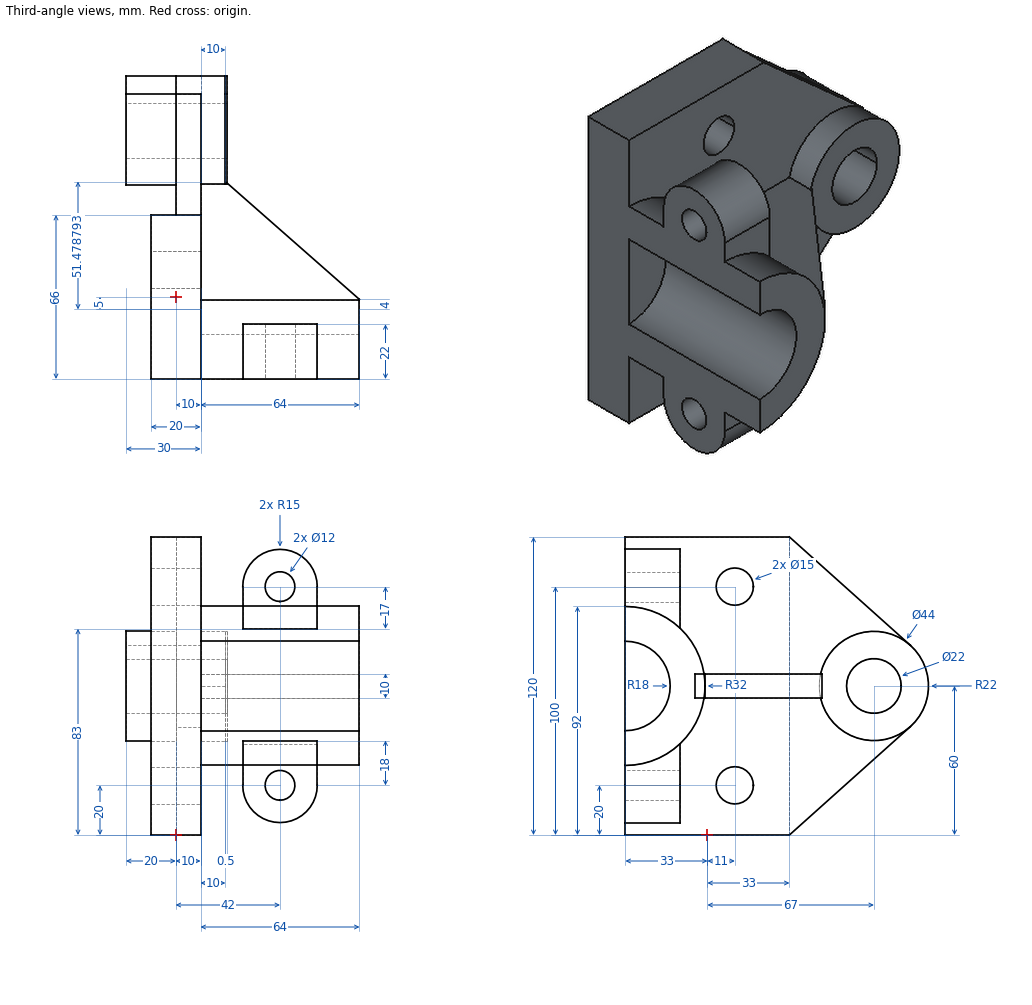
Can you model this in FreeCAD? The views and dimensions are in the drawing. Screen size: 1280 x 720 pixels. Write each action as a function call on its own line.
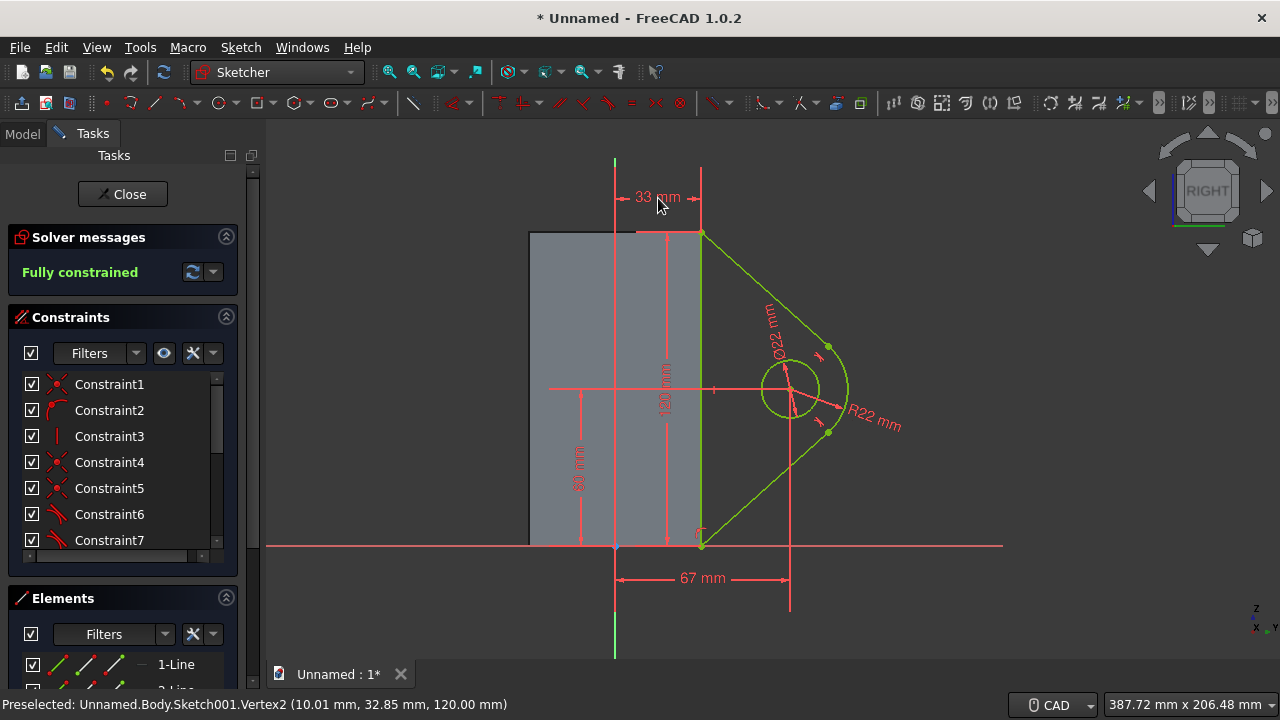
click(123, 194)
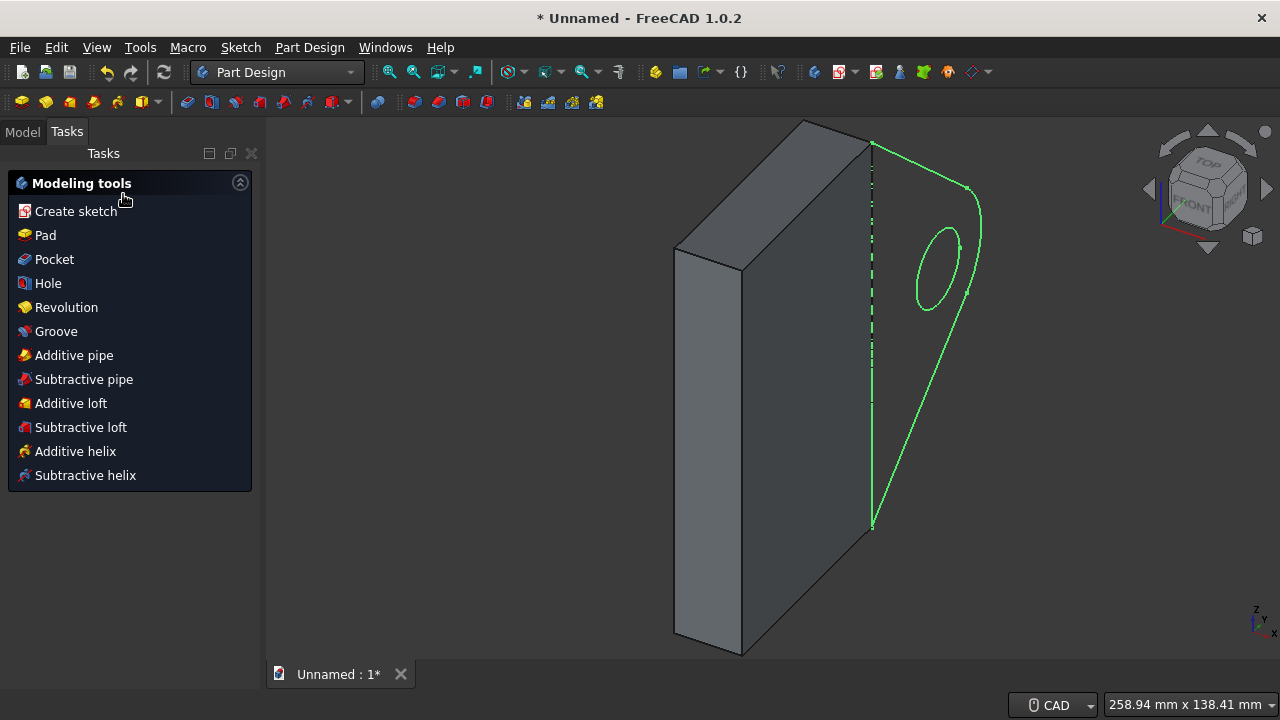
click(22, 102)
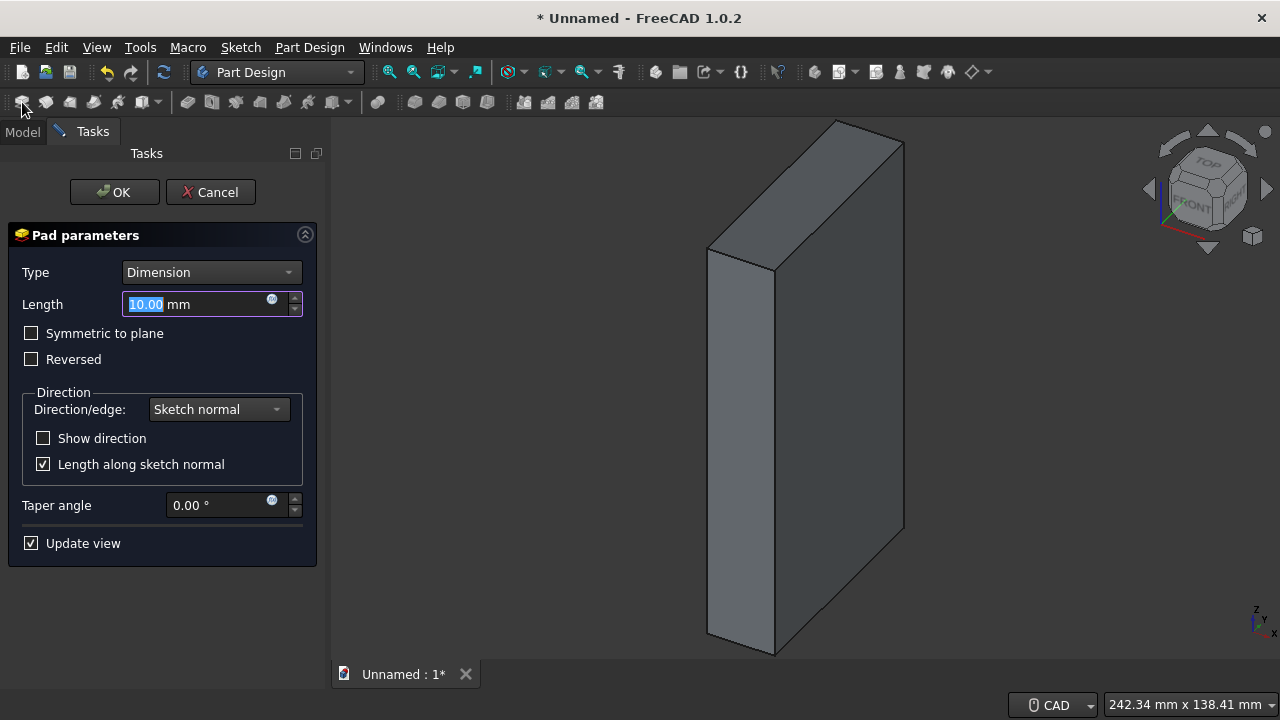
text(10)
key(Tab)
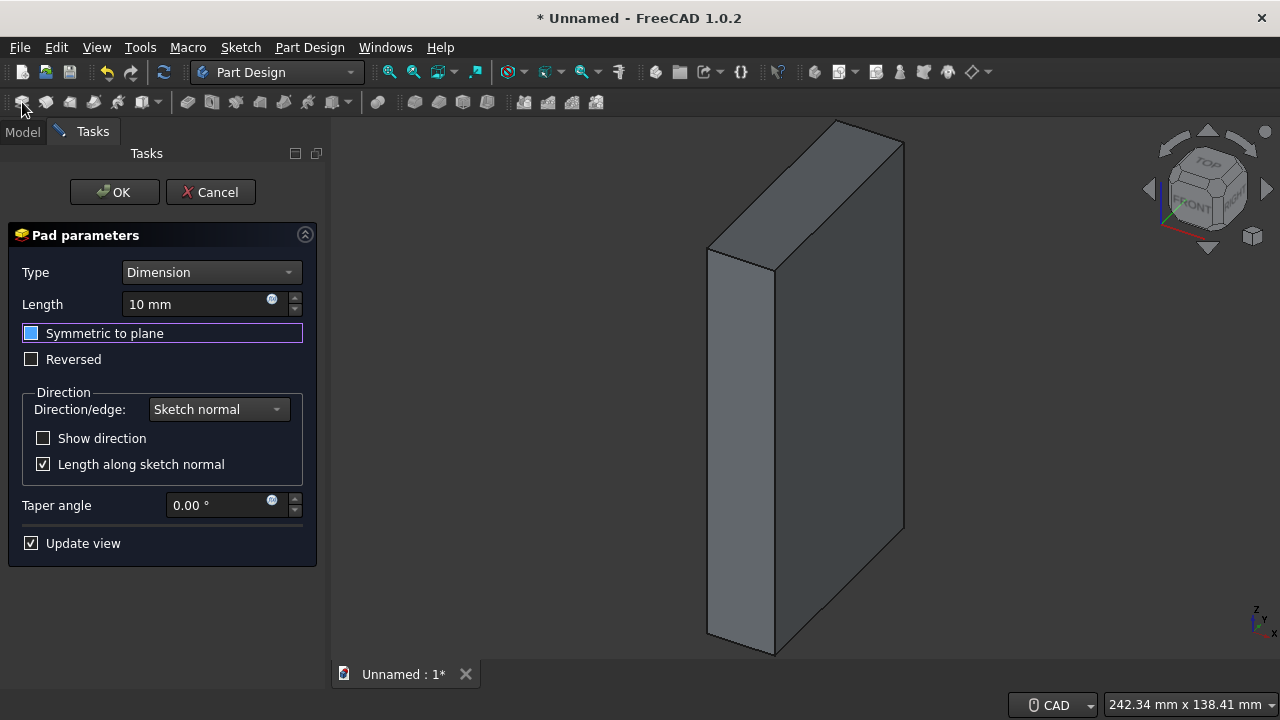
click(30, 359)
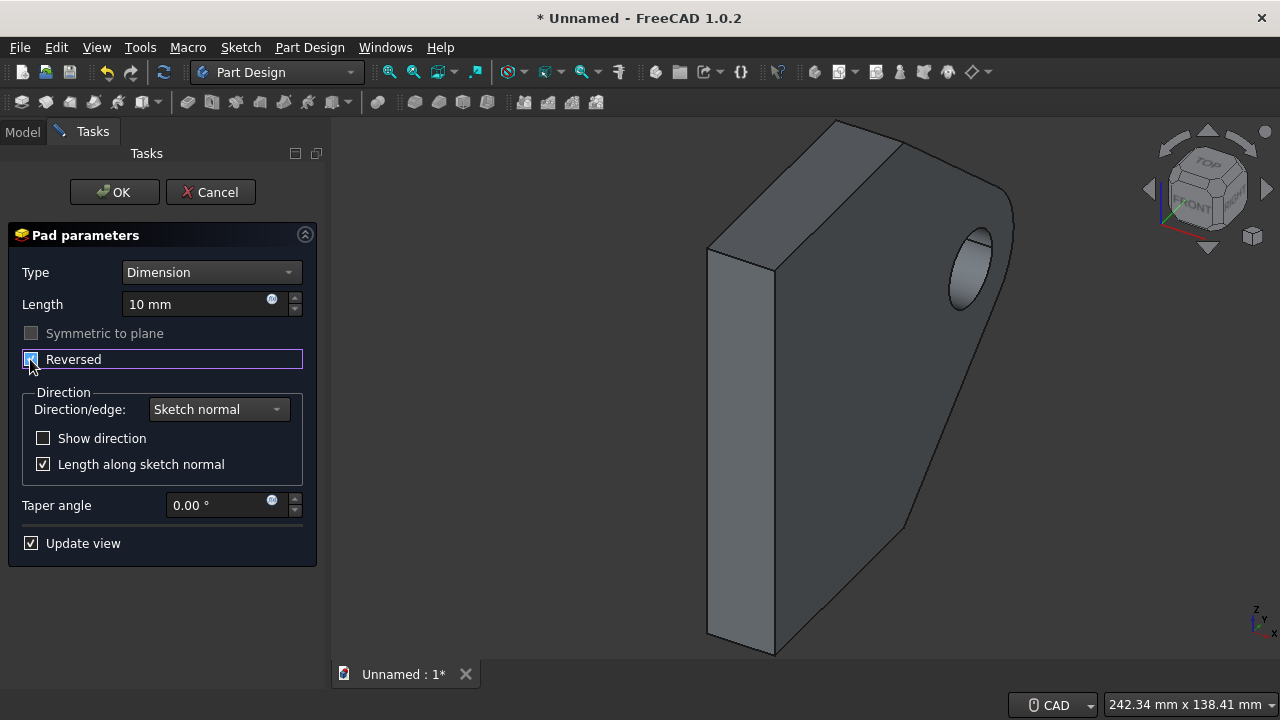
click(115, 192)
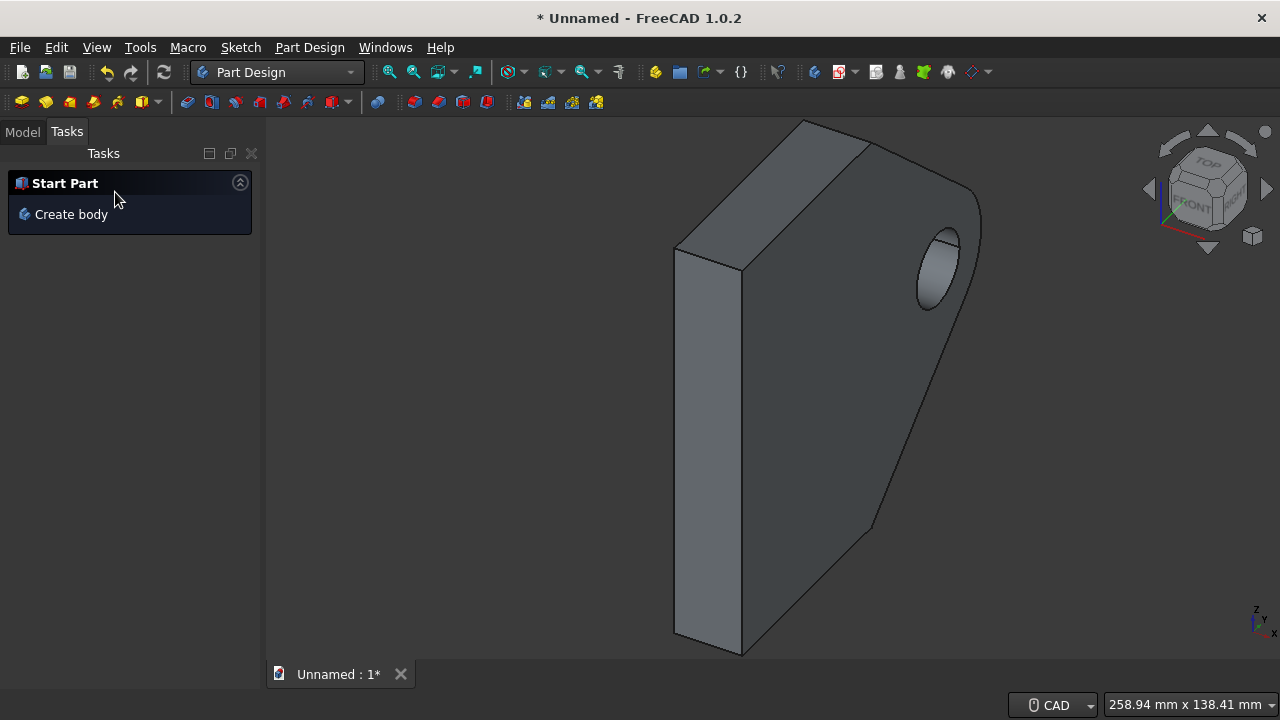
click(390, 72)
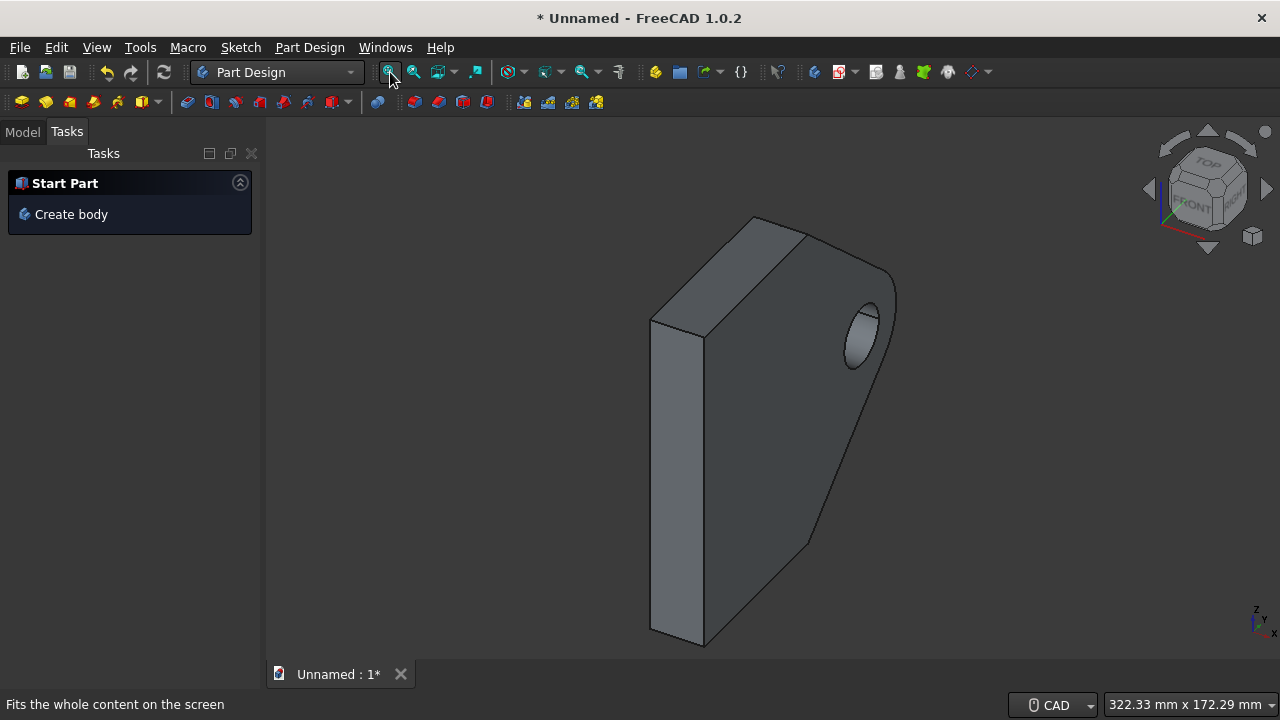
key(6)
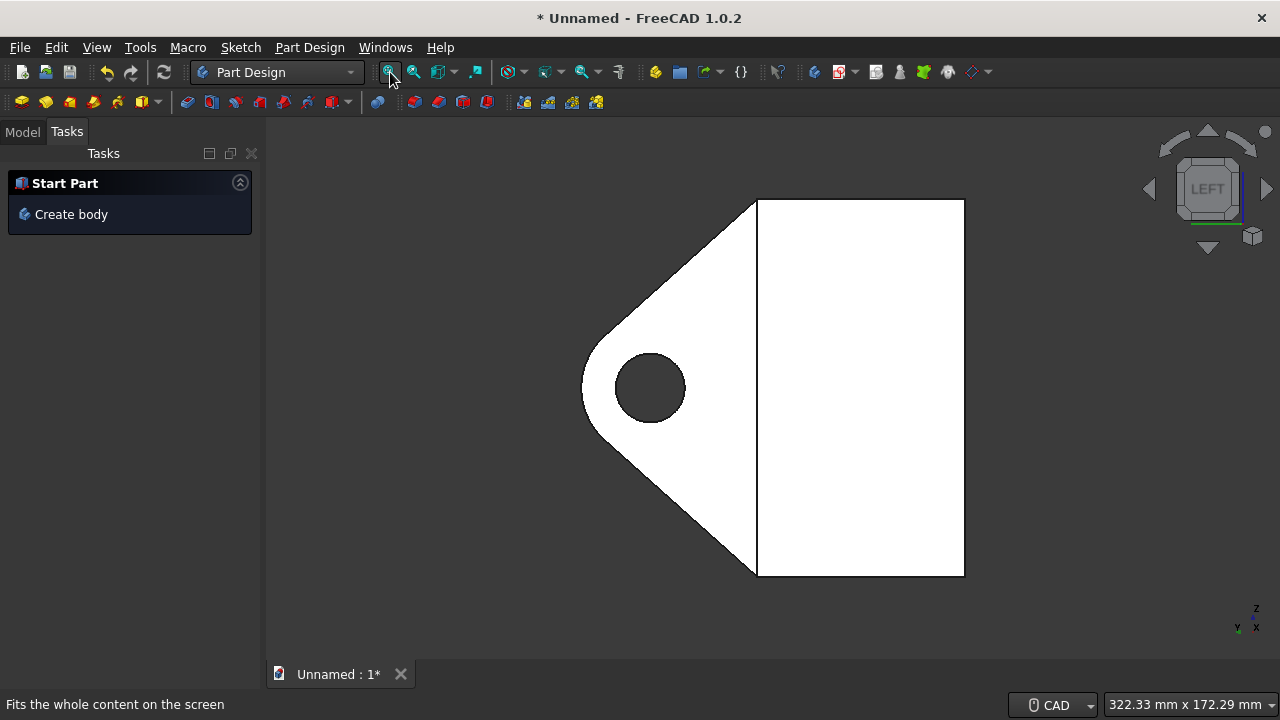
click(720, 333)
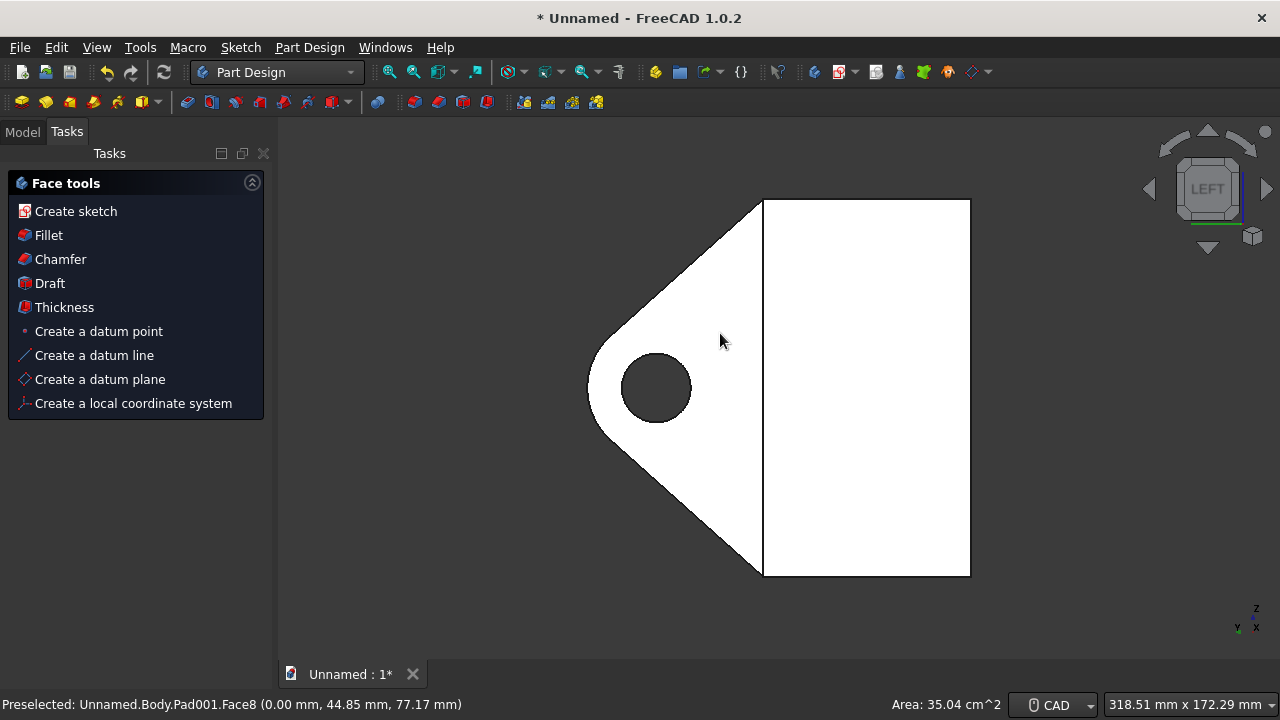
click(840, 72)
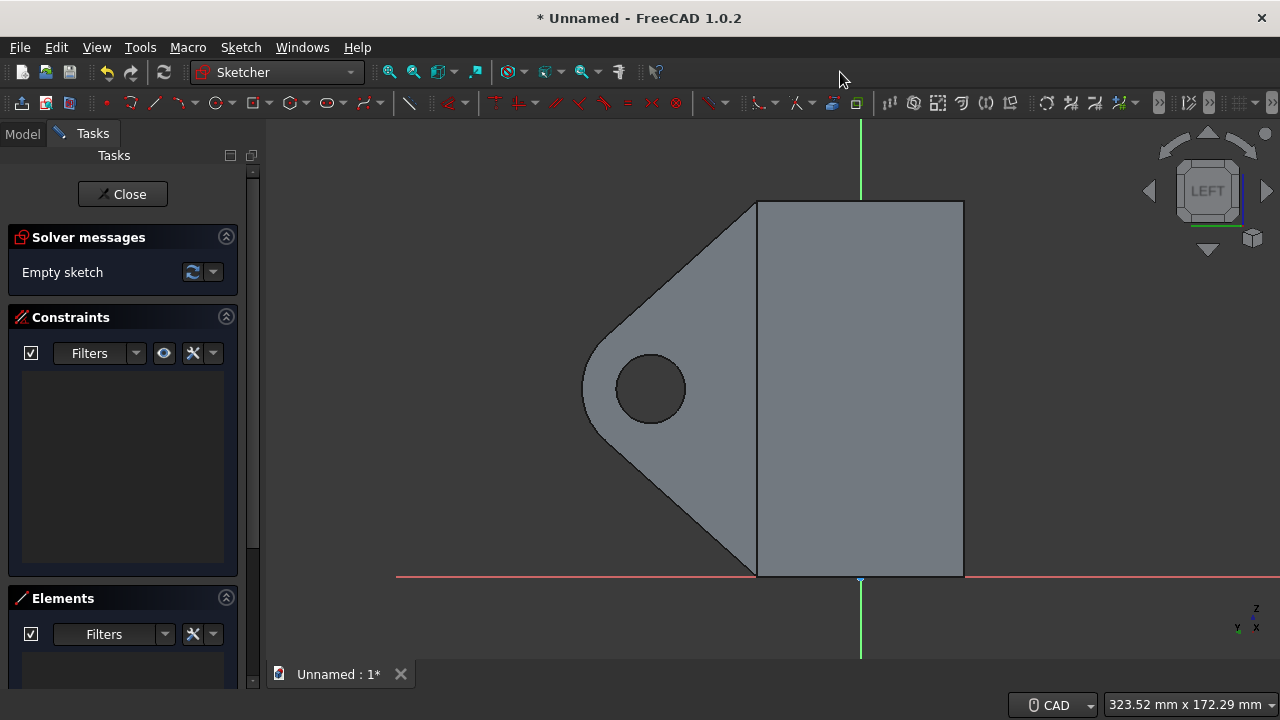
click(70, 104)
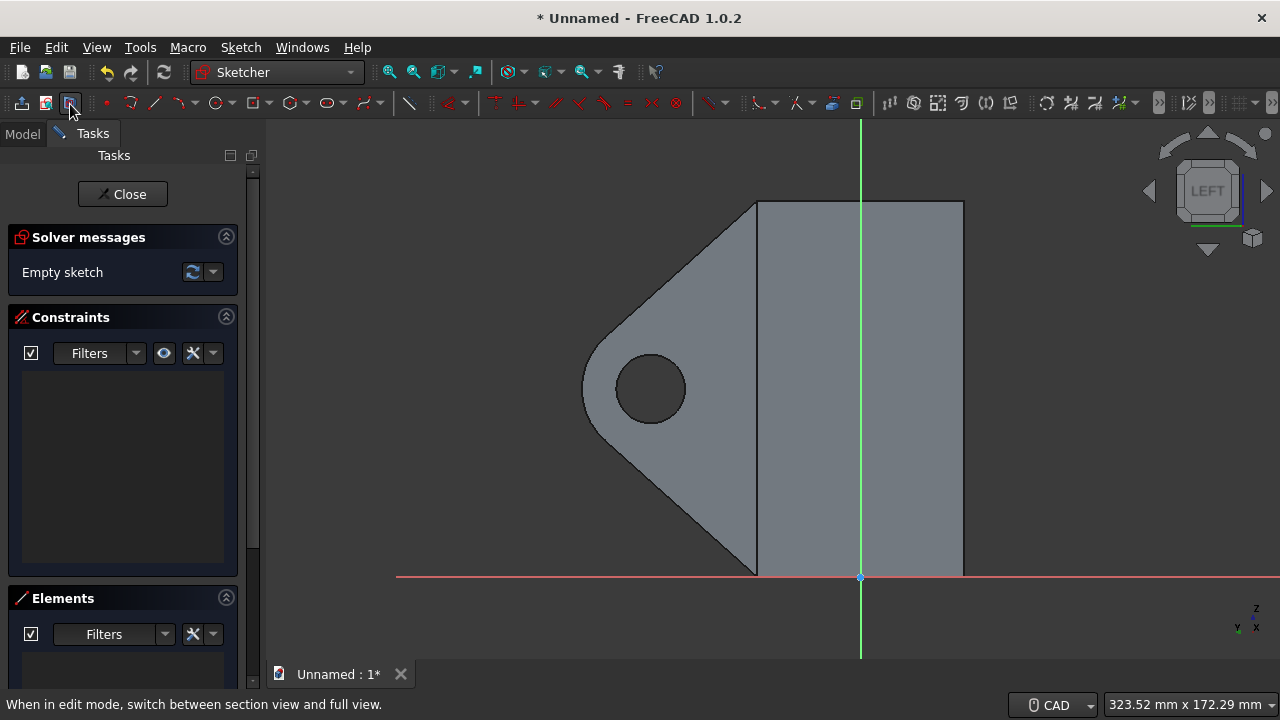
click(216, 104)